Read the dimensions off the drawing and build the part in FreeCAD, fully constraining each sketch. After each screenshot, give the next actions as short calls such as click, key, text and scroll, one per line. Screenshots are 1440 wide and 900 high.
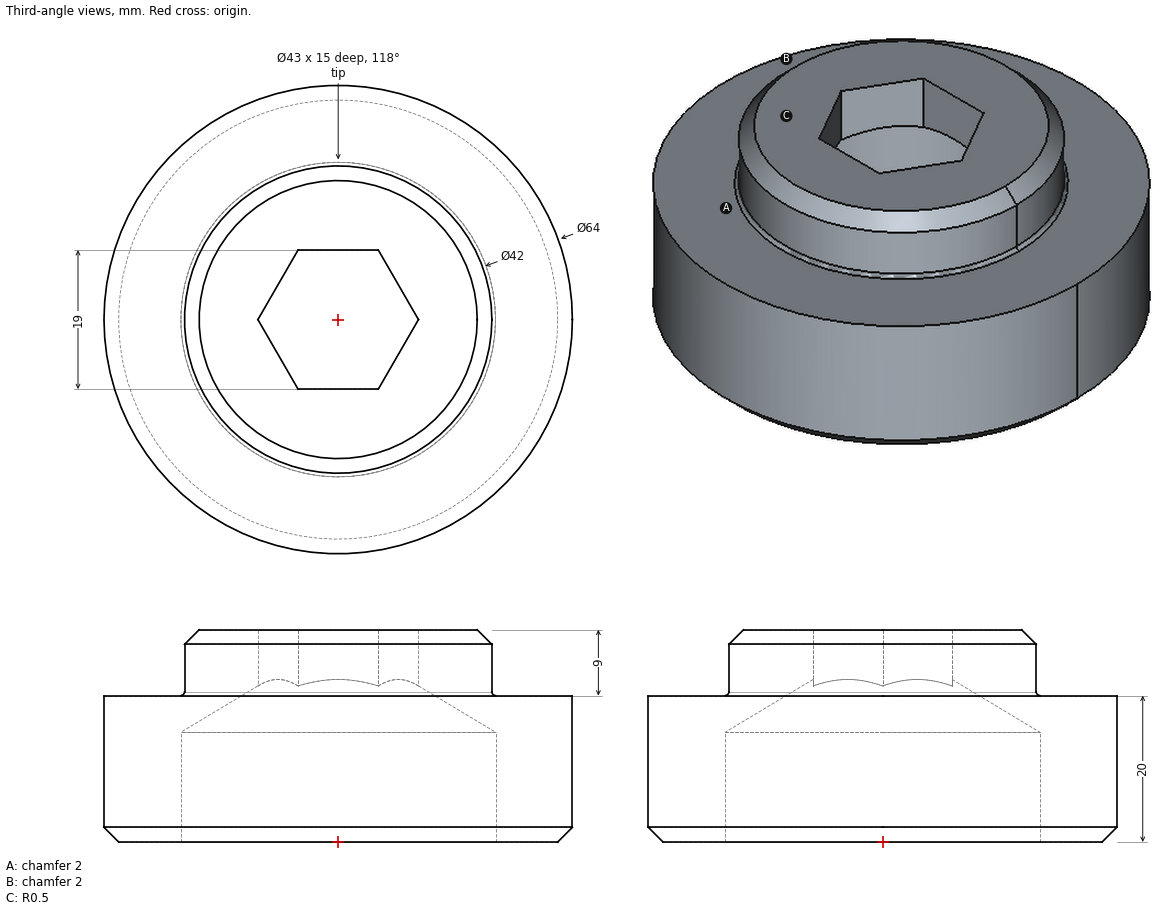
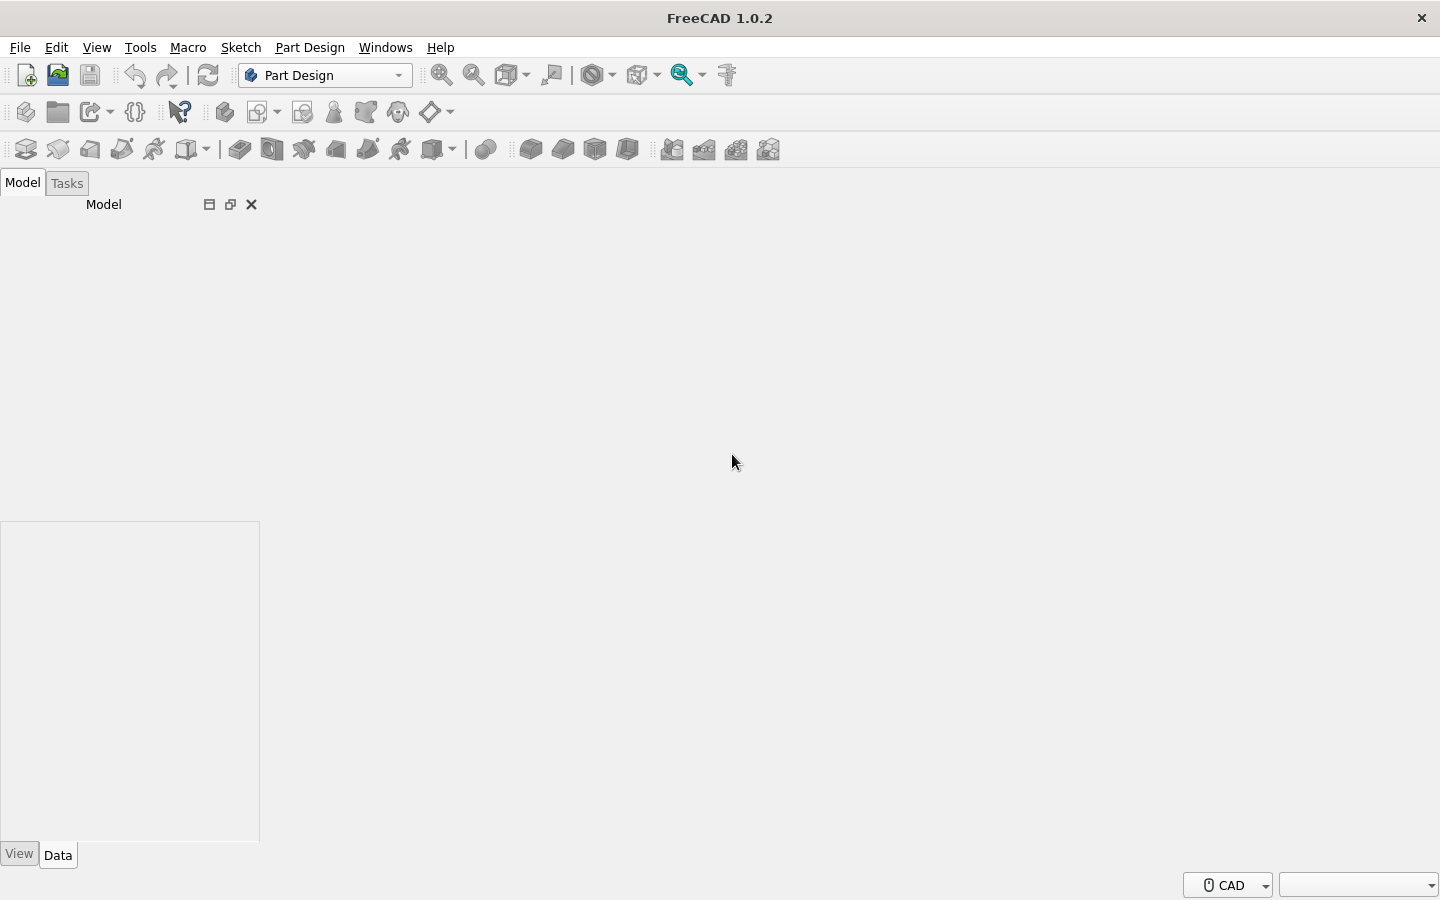
click(26, 76)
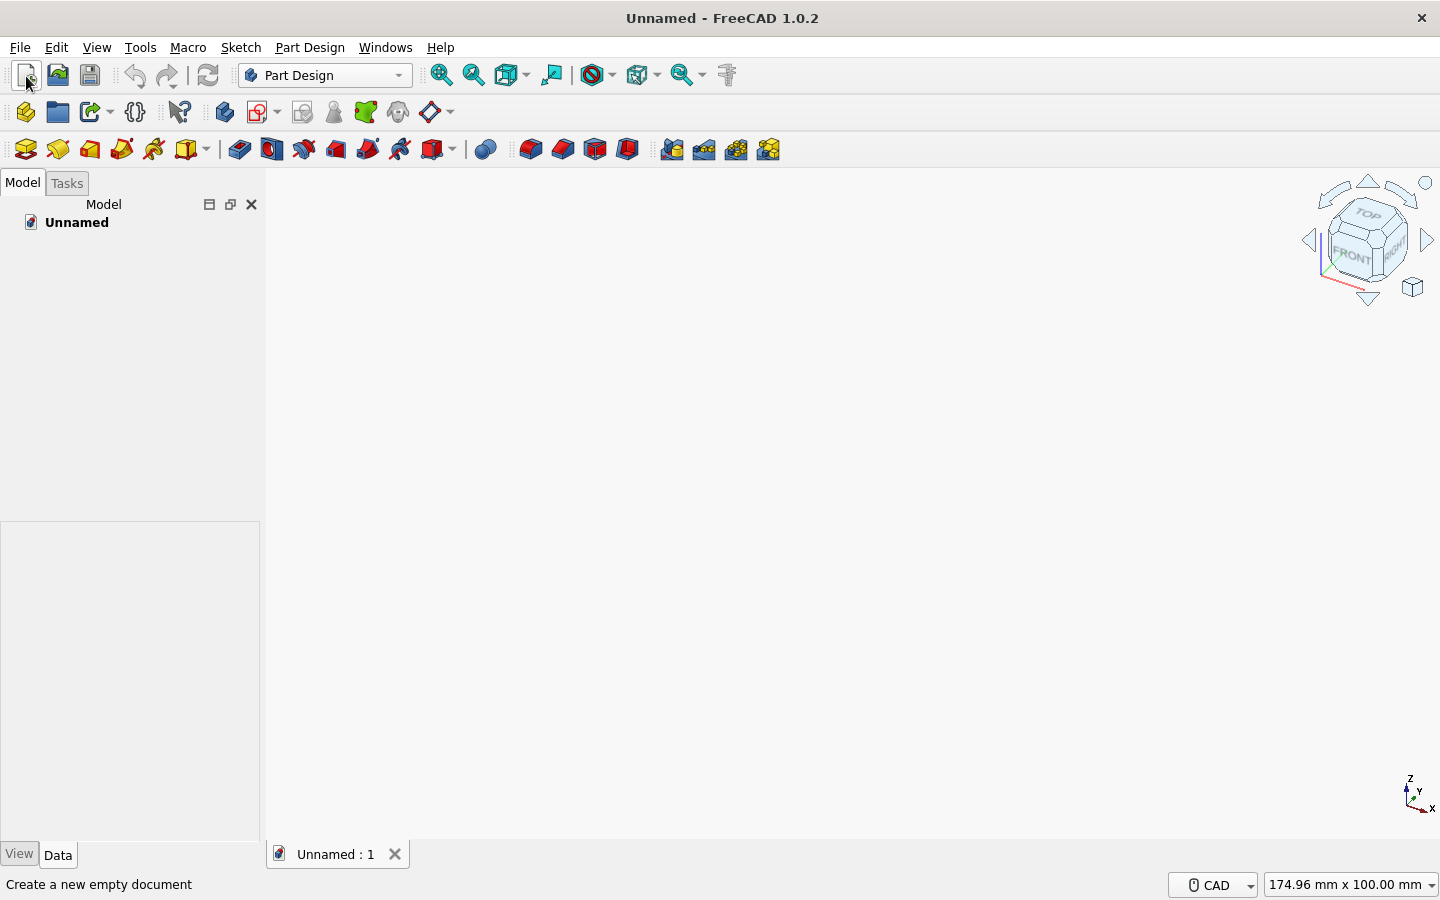
click(258, 112)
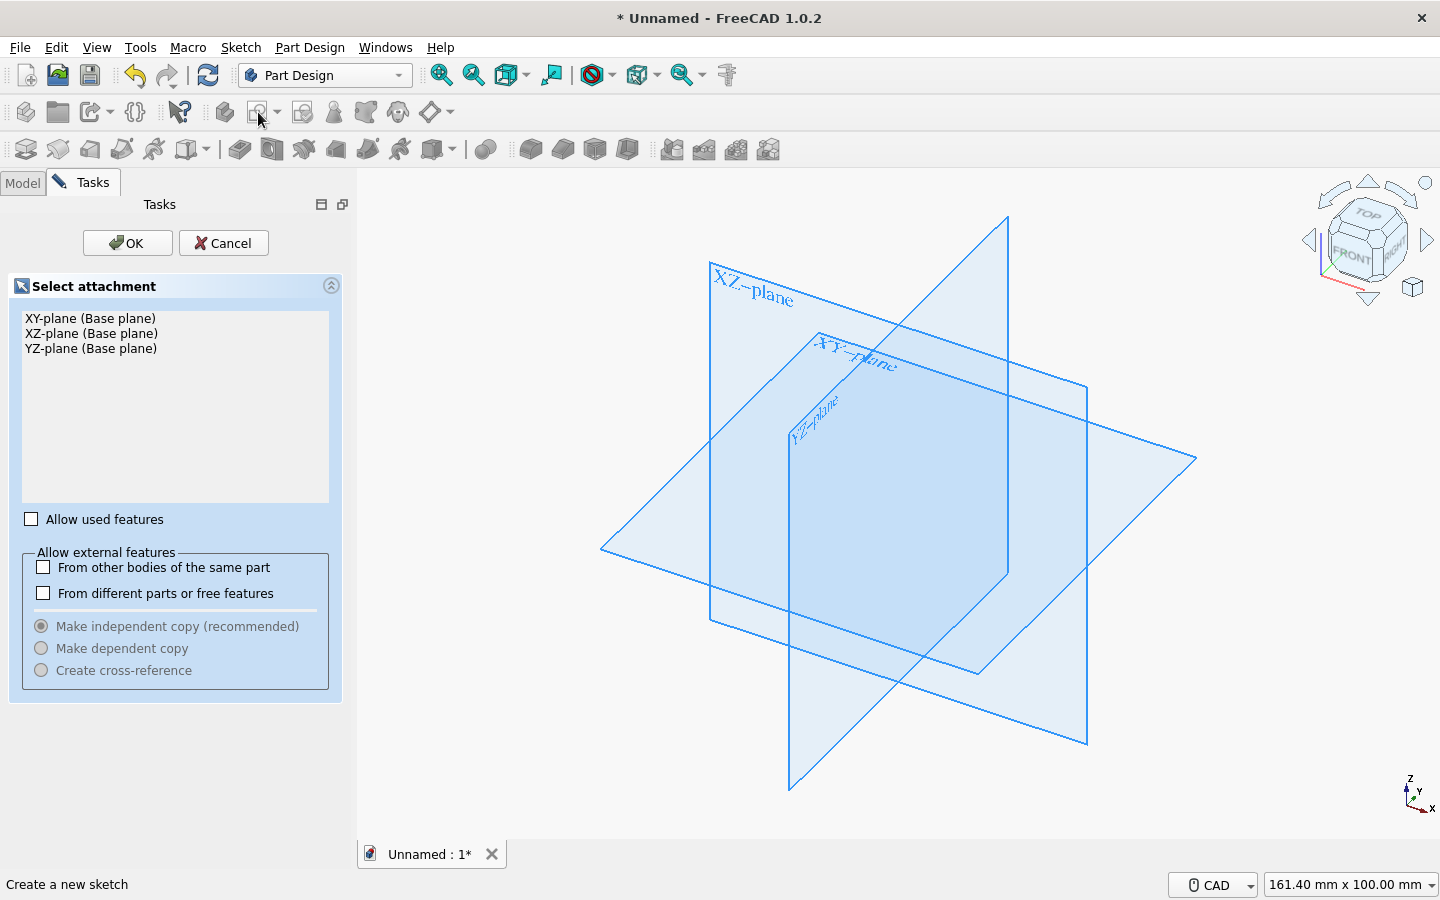
click(82, 318)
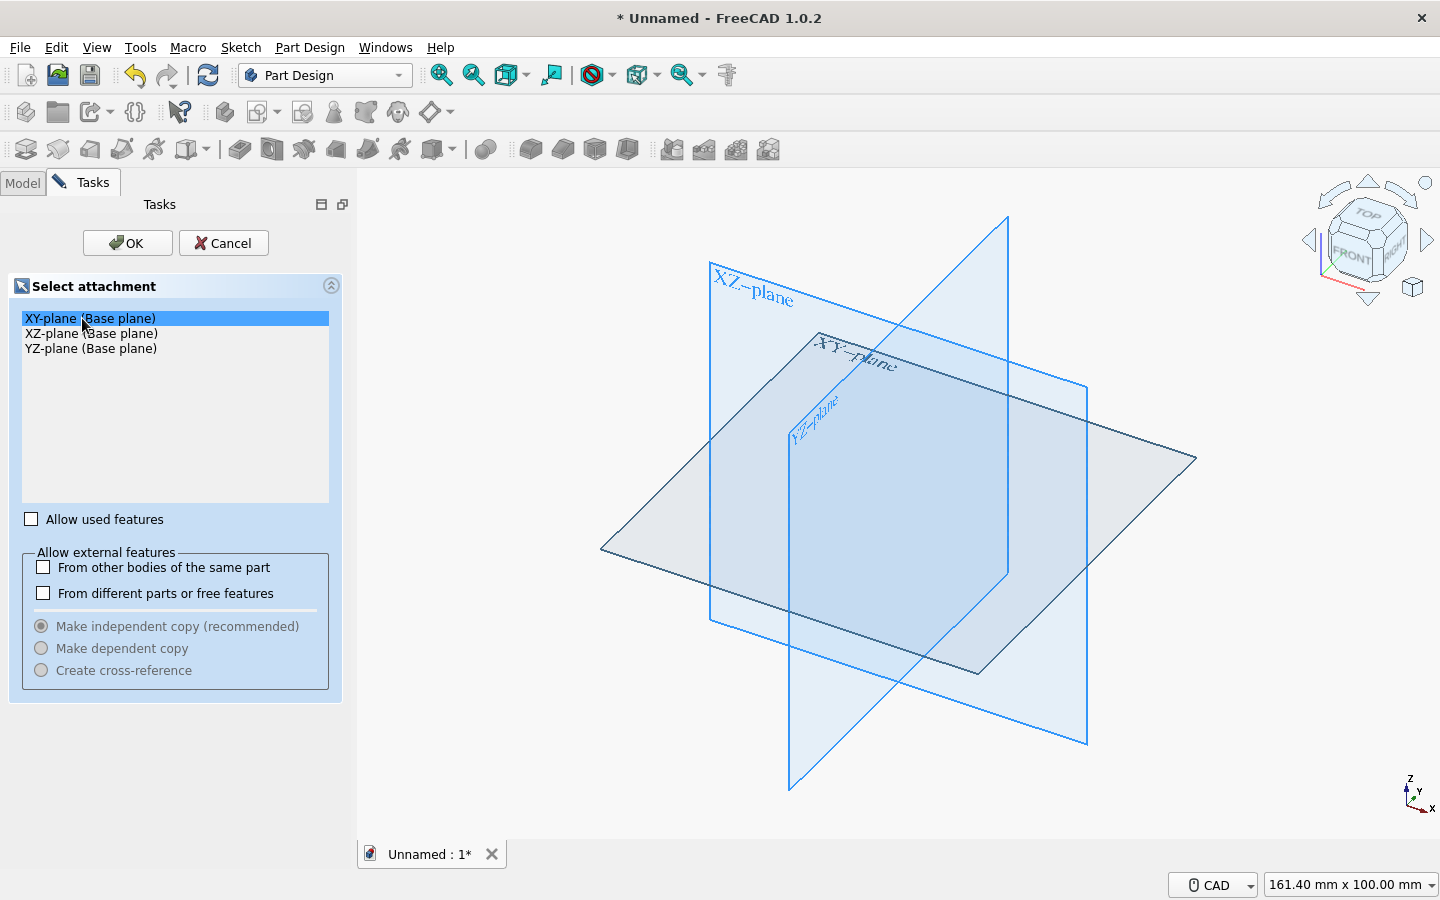
click(128, 243)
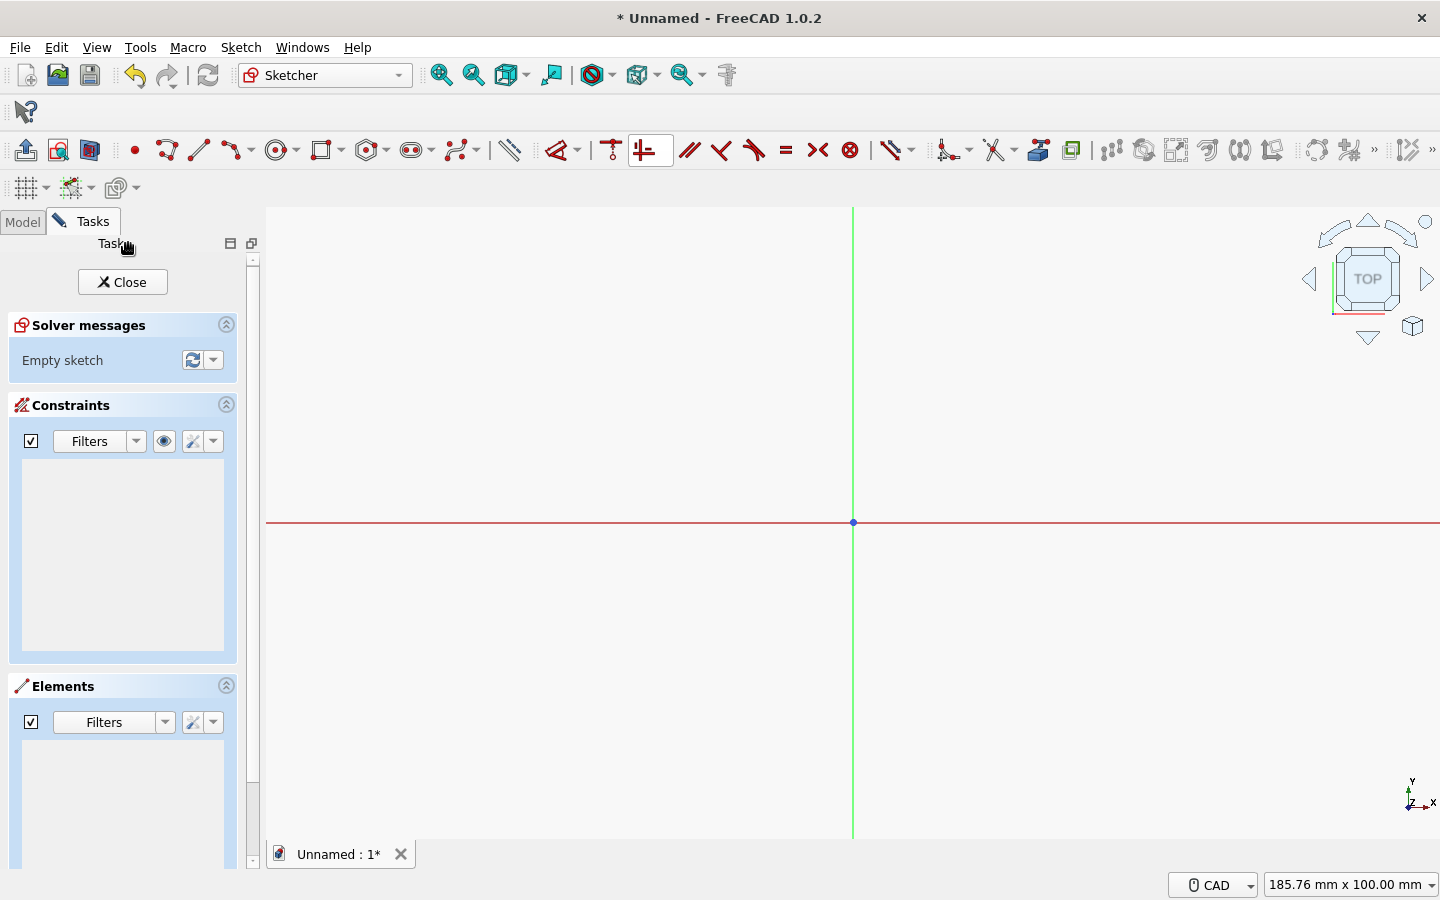
click(276, 150)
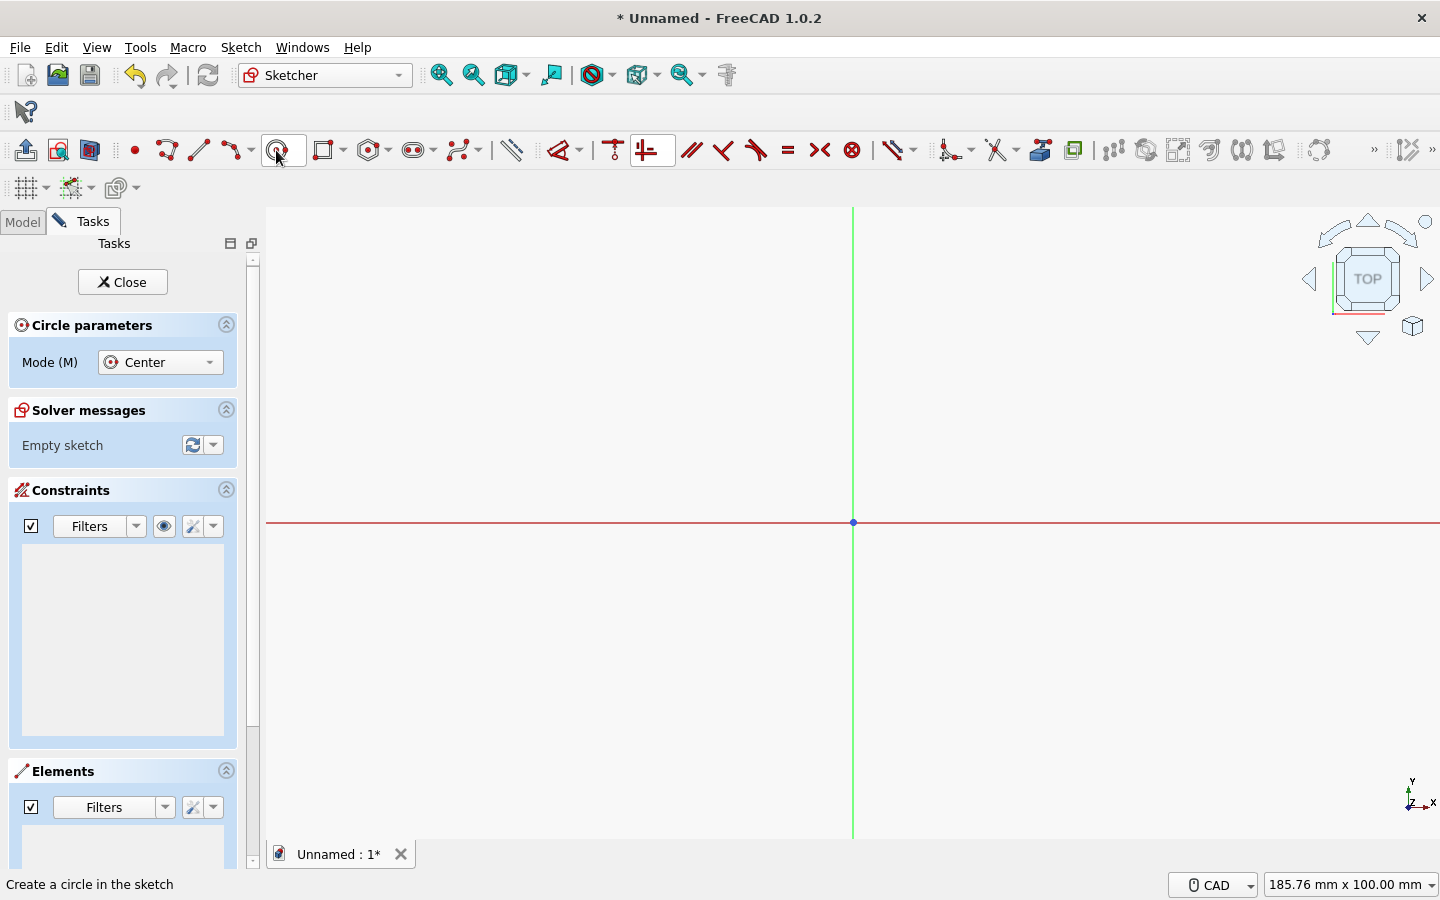
click(853, 523)
move(996, 380)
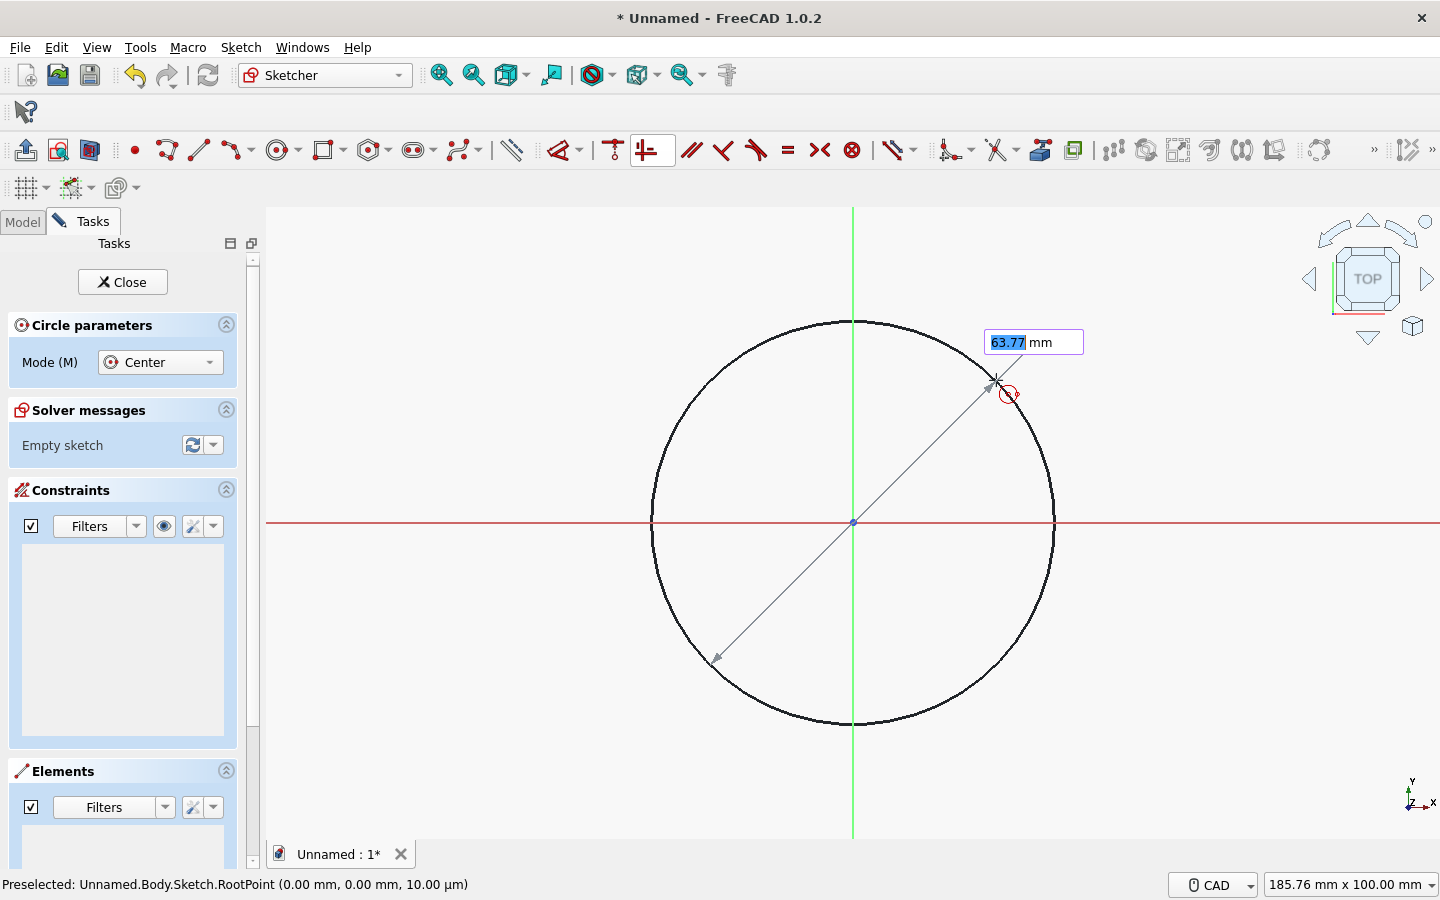
text(64)
key(Return)
key(Escape)